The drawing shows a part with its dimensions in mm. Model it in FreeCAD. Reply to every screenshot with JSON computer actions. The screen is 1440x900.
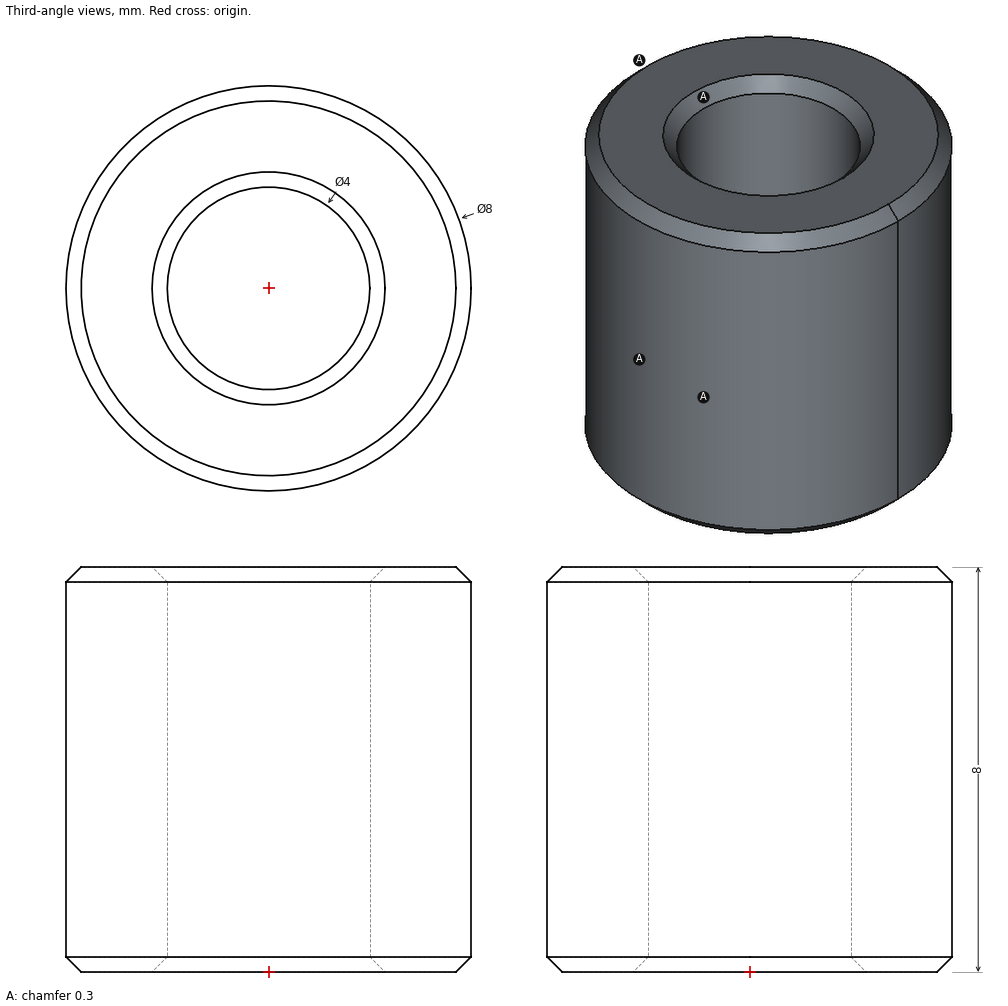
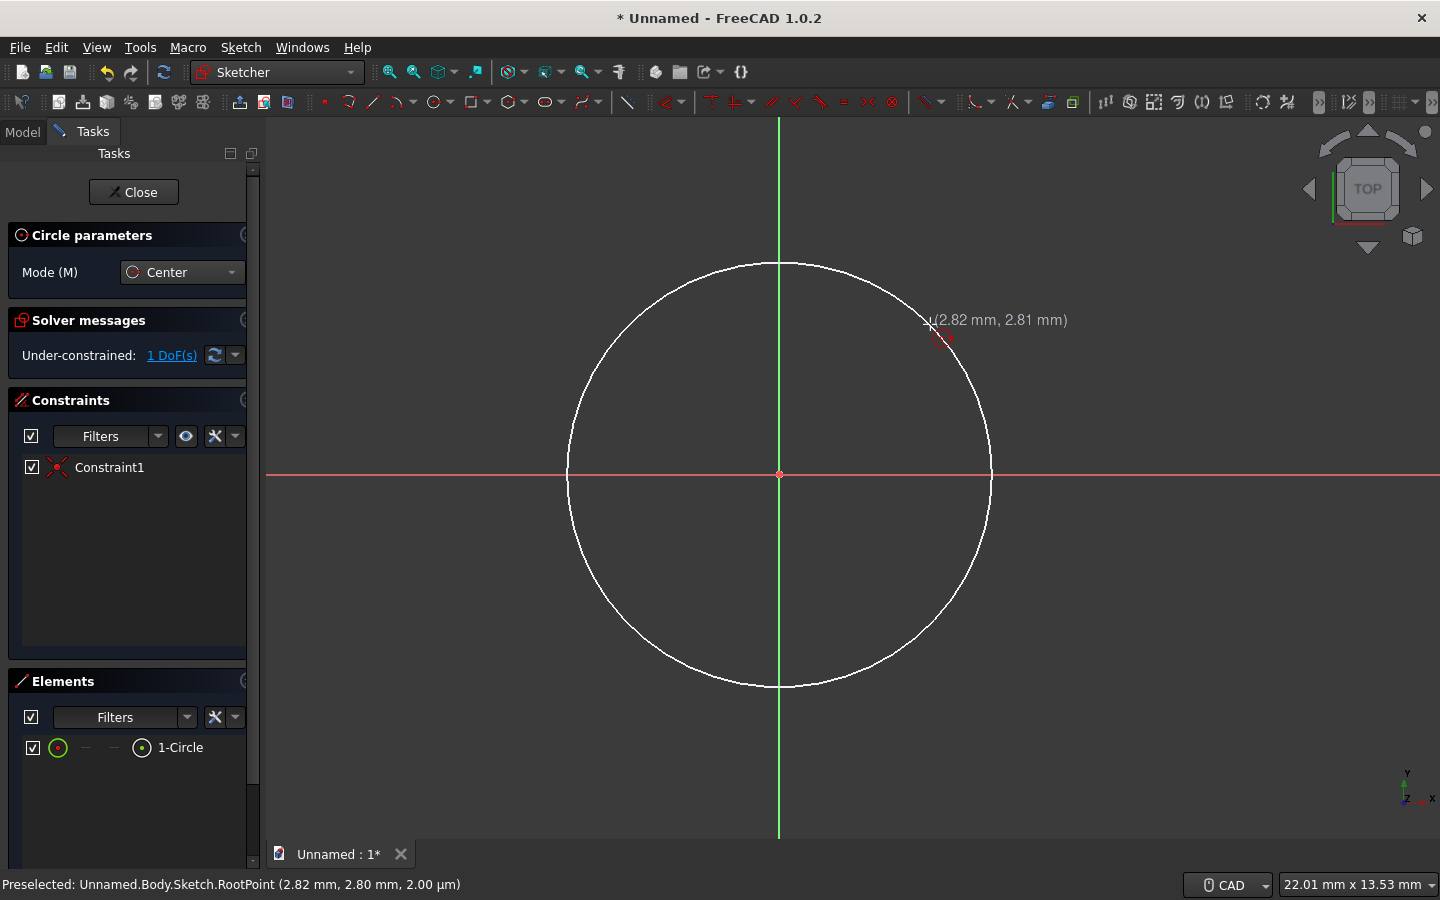
{"action": "left_click", "coordinate": [779, 475]}
{"action": "left_click", "coordinate": [855, 399]}
{"action": "key", "text": "Escape"}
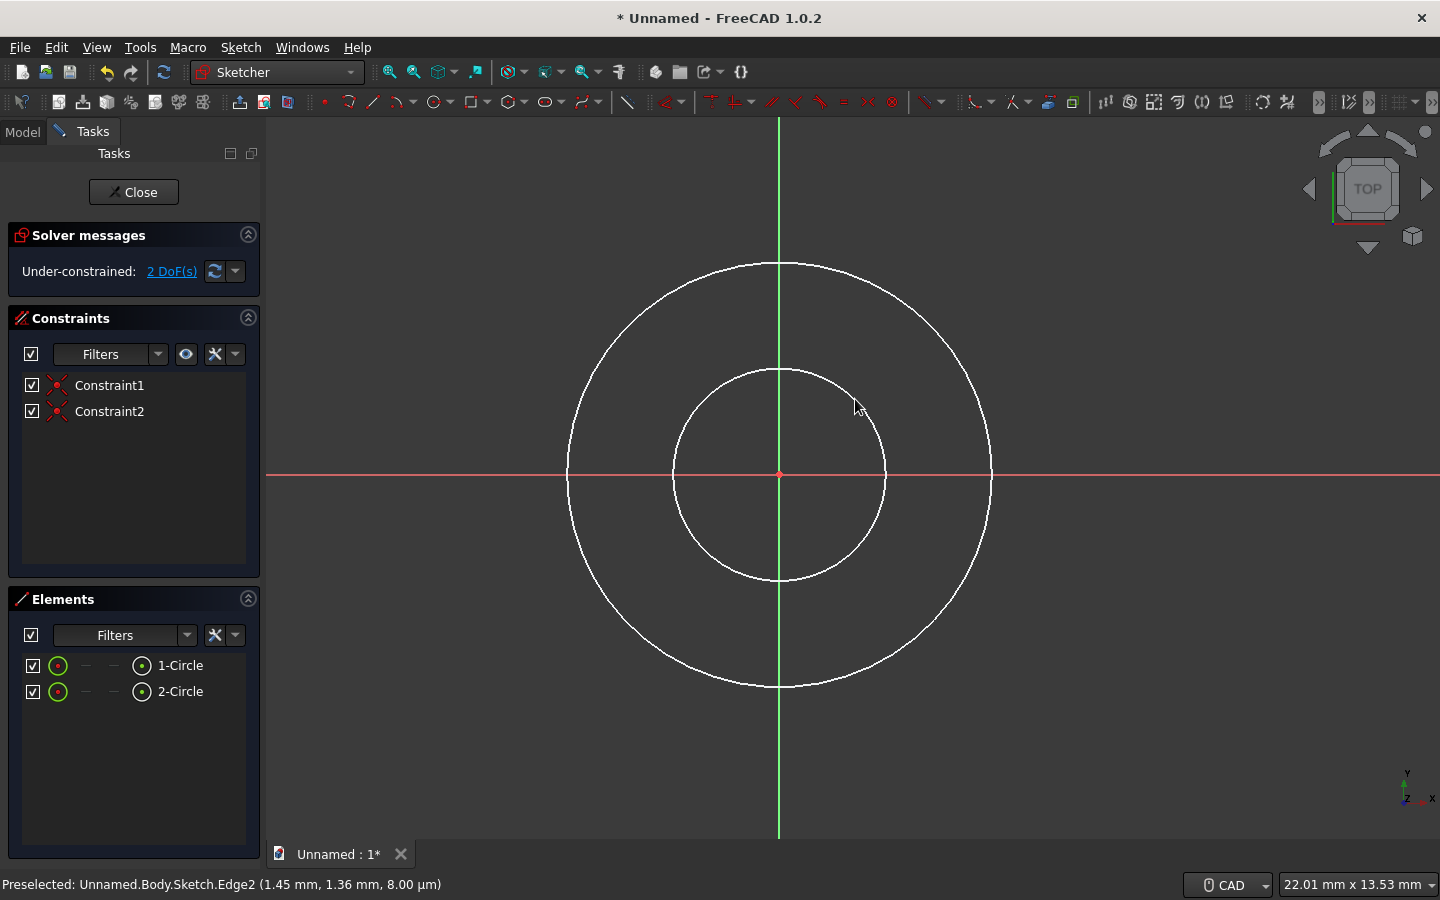
{"action": "key", "text": "d"}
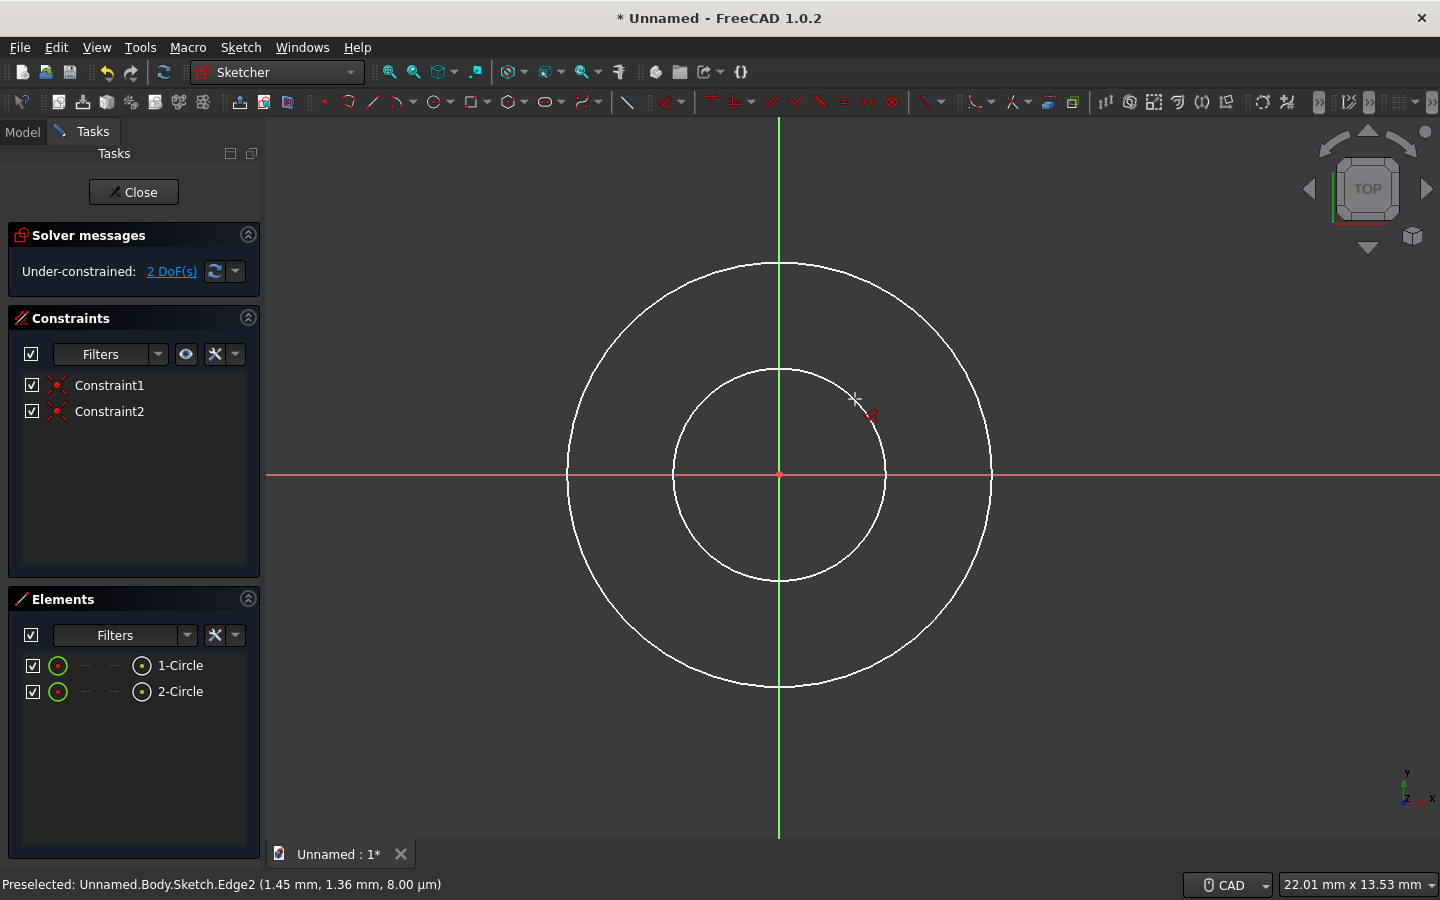
{"action": "left_click", "coordinate": [929, 324]}
{"action": "left_click", "coordinate": [952, 301]}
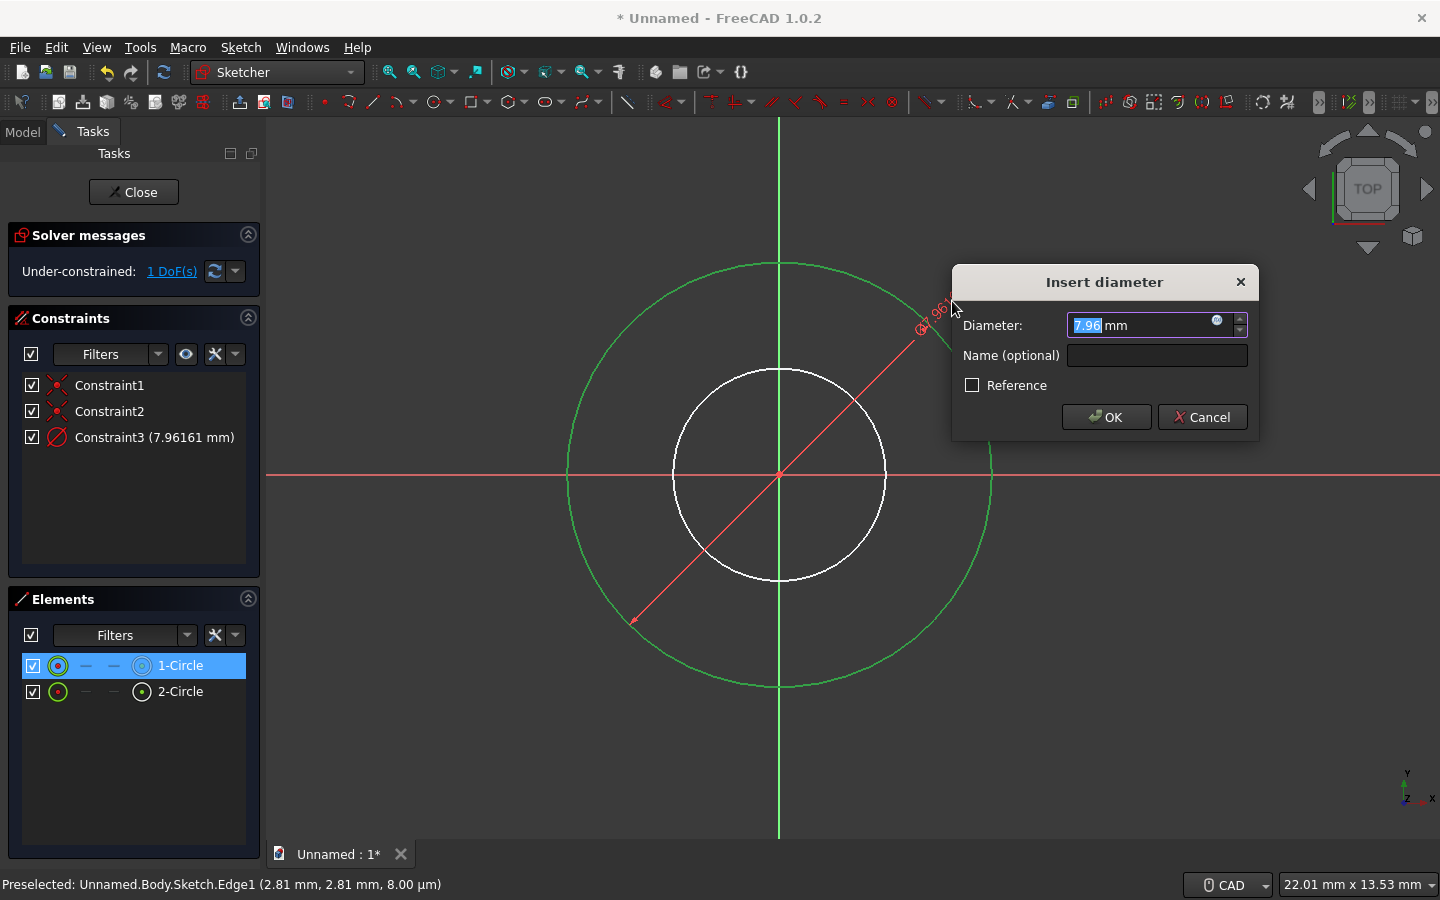
{"action": "type", "text": "8"}
{"action": "key", "text": "Return"}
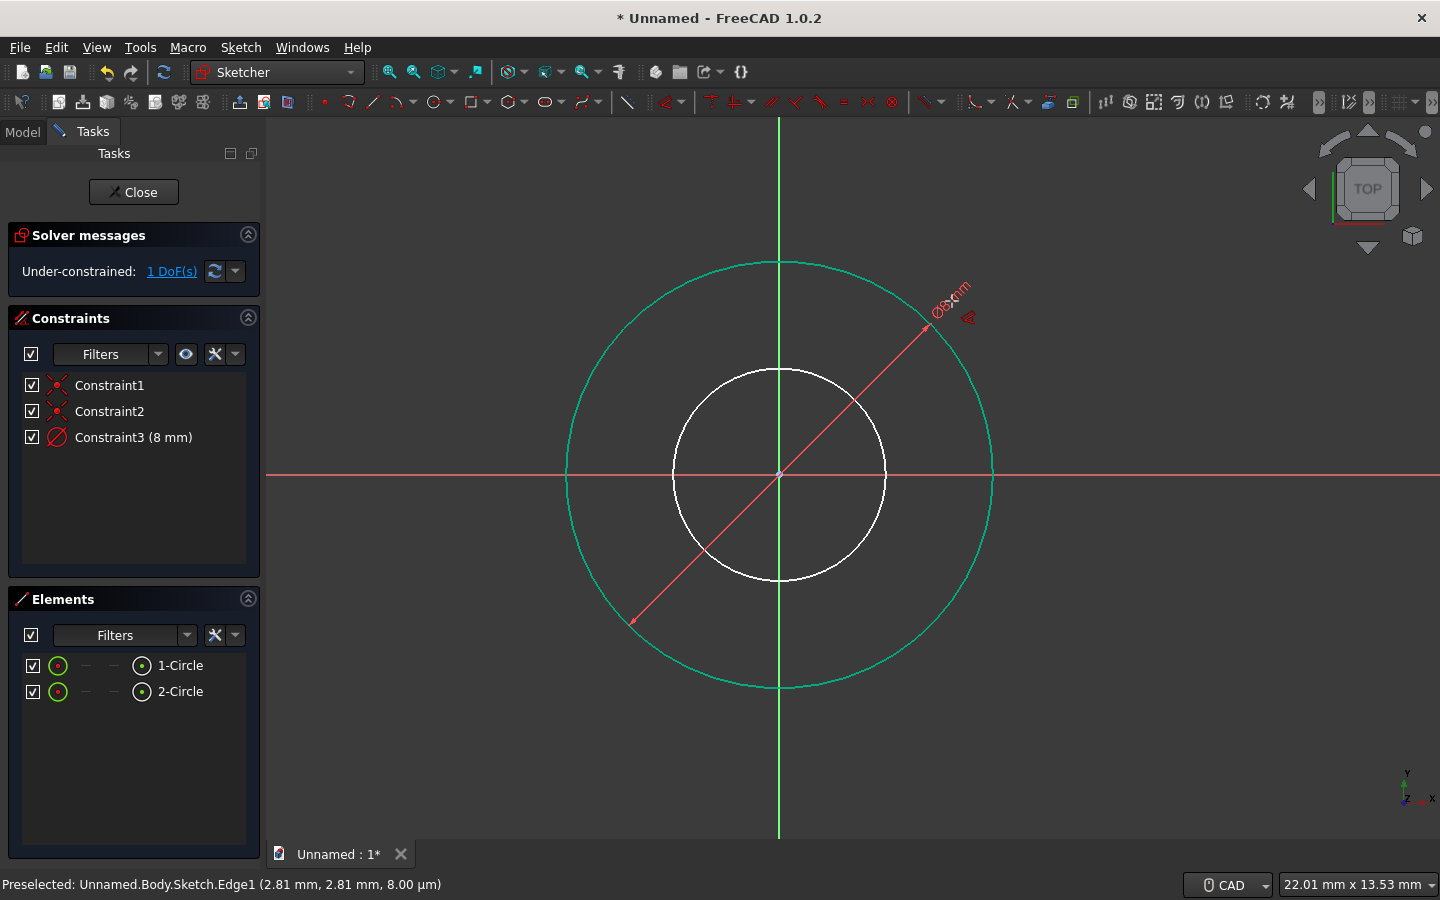
{"action": "left_click", "coordinate": [854, 399]}
{"action": "left_click", "coordinate": [876, 376]}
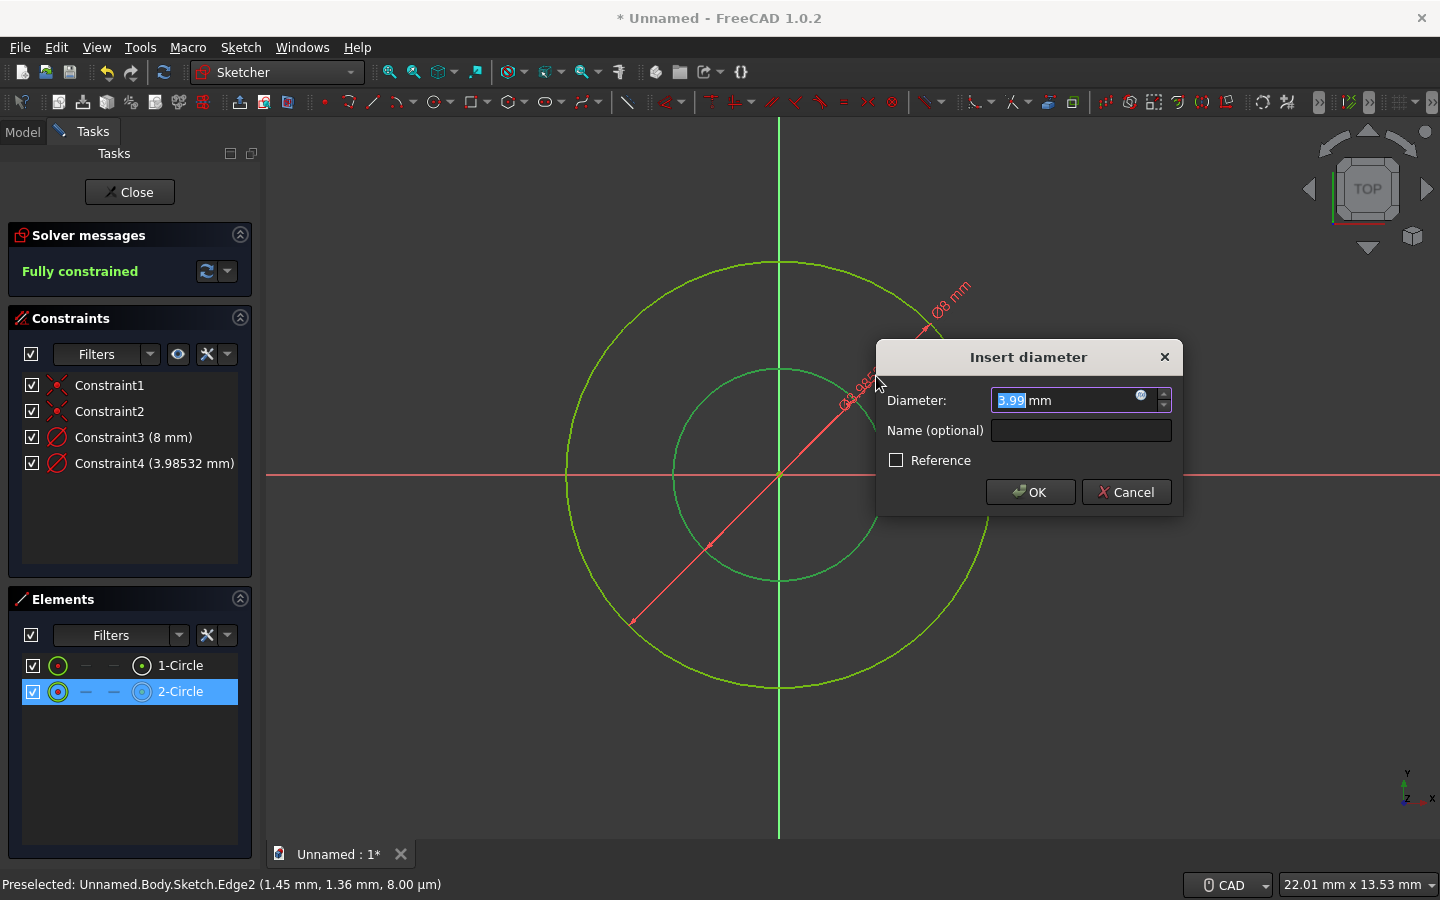
{"action": "type", "text": "4"}
{"action": "key", "text": "Return"}
{"action": "key", "text": "Escape"}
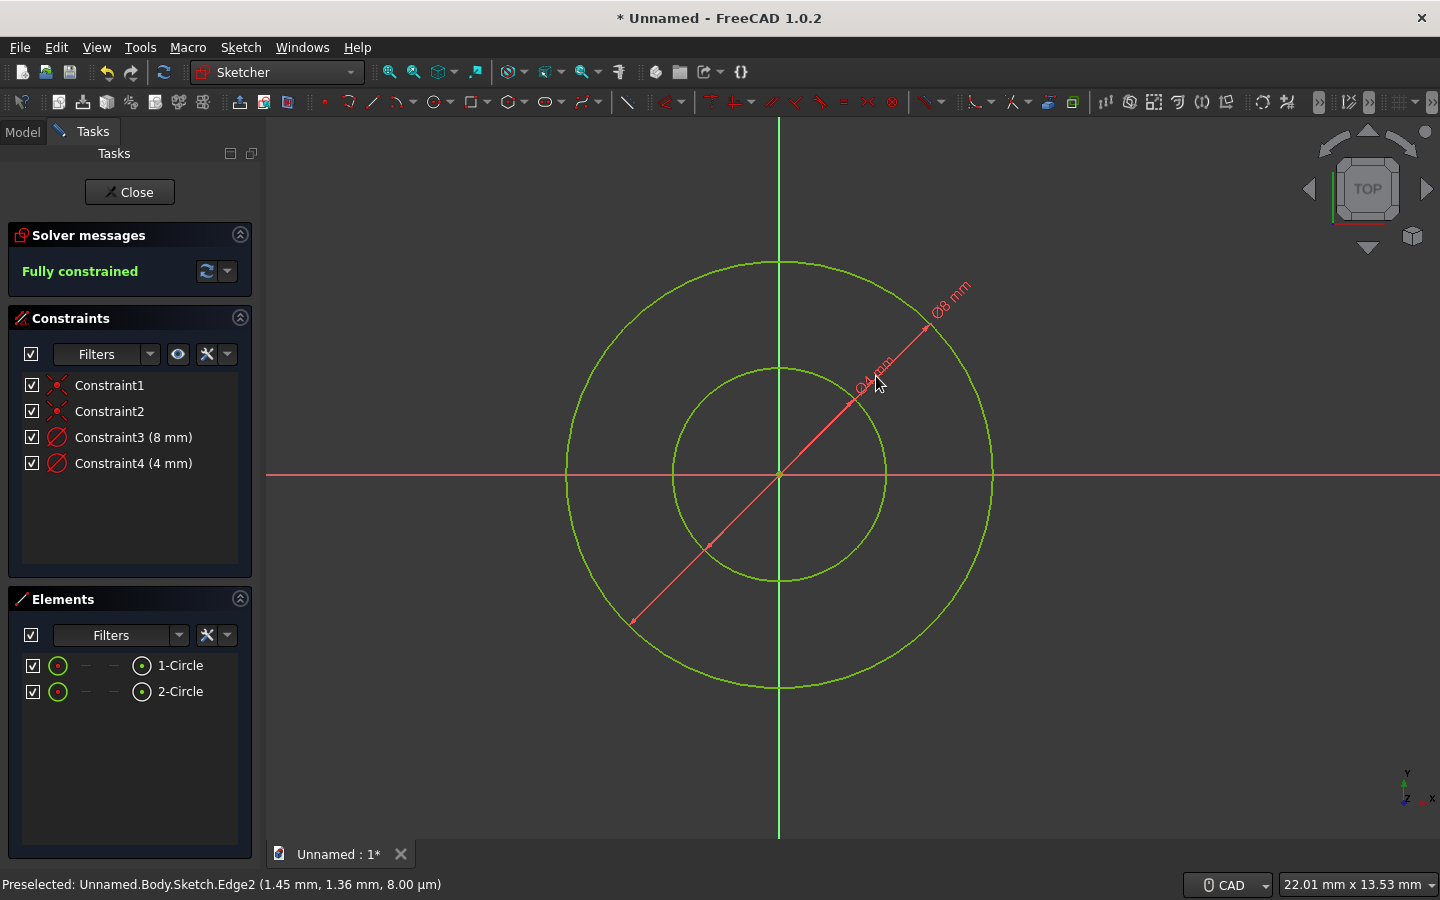
{"action": "left_click", "coordinate": [130, 192]}